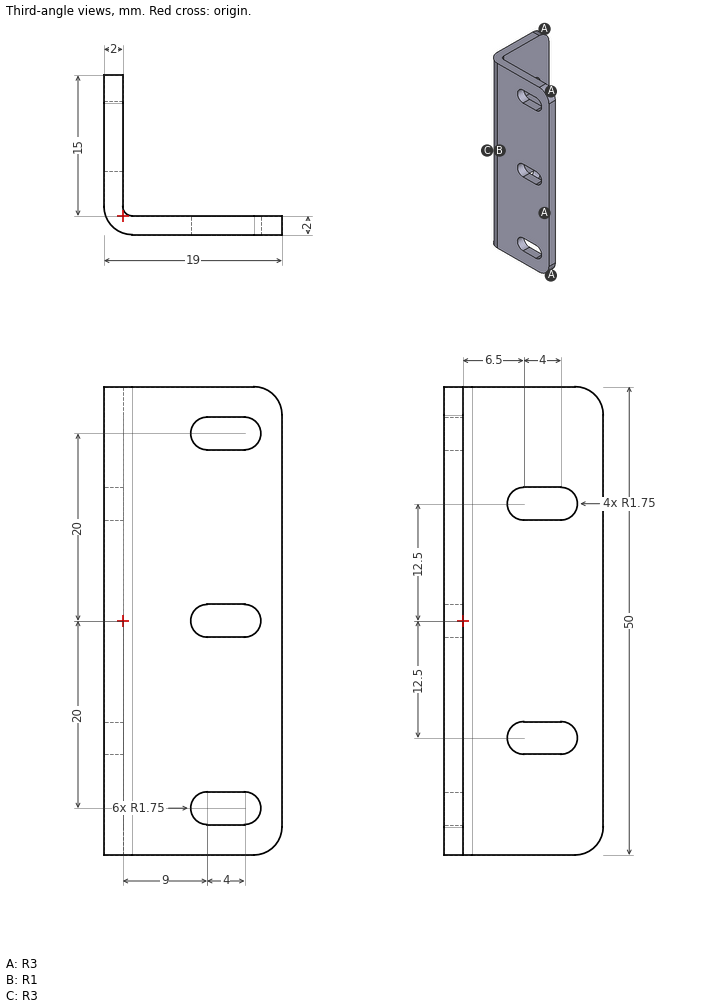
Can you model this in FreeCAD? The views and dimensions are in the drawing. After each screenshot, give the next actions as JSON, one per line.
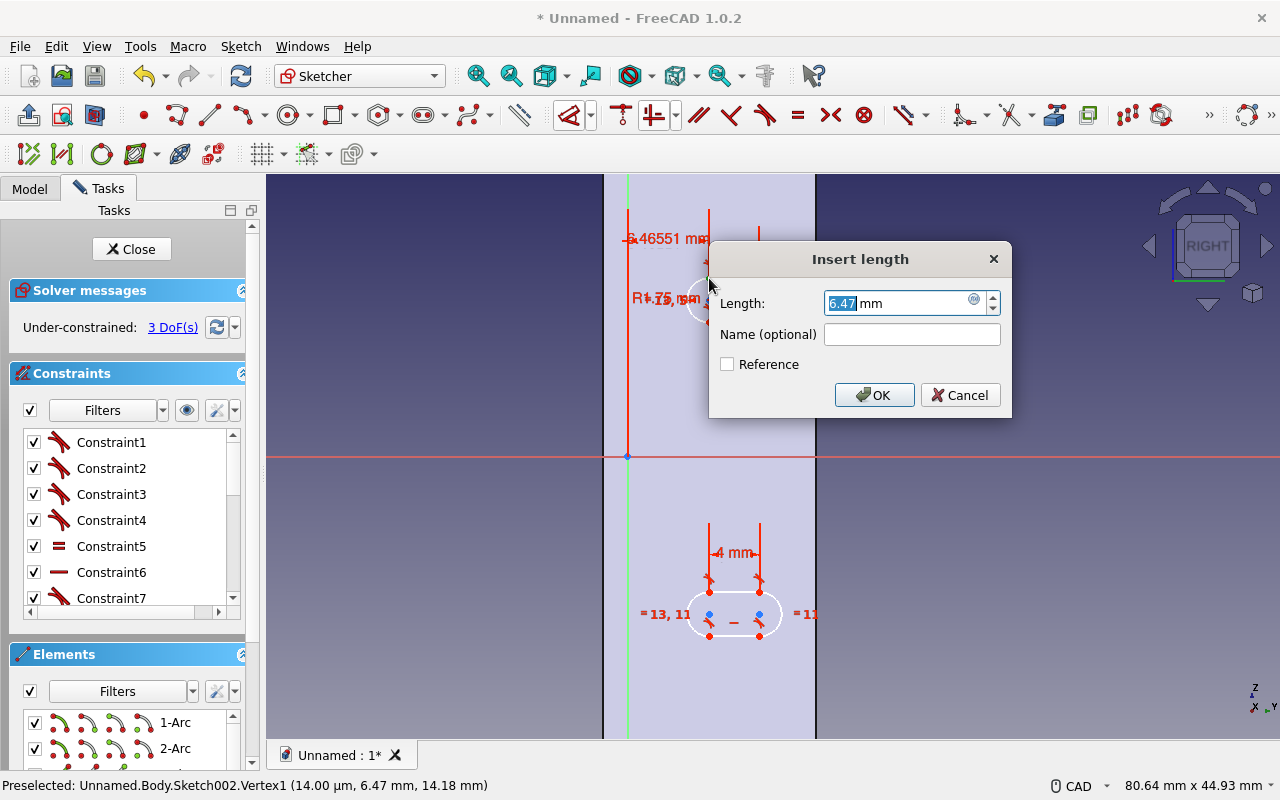
{"action": "type", "text": "6.5"}
{"action": "key", "text": "Return"}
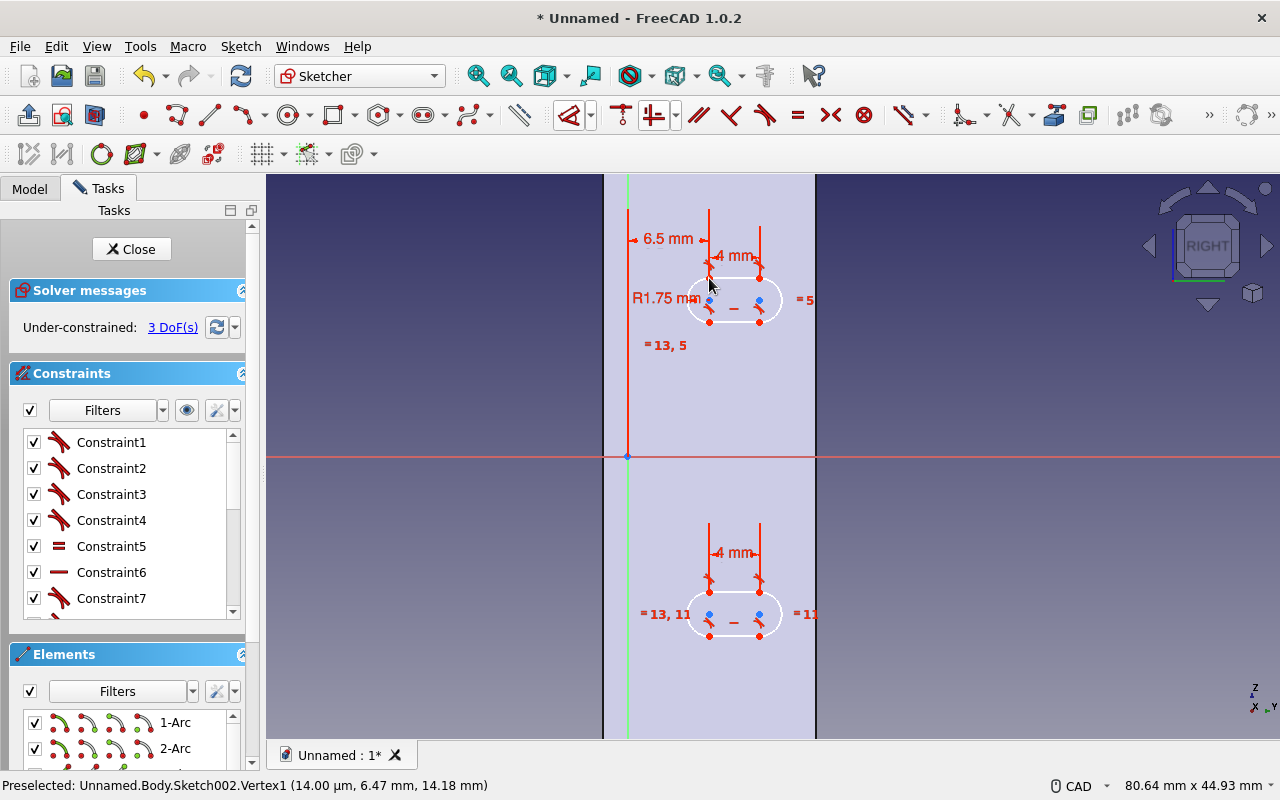
{"action": "left_click", "coordinate": [709, 592]}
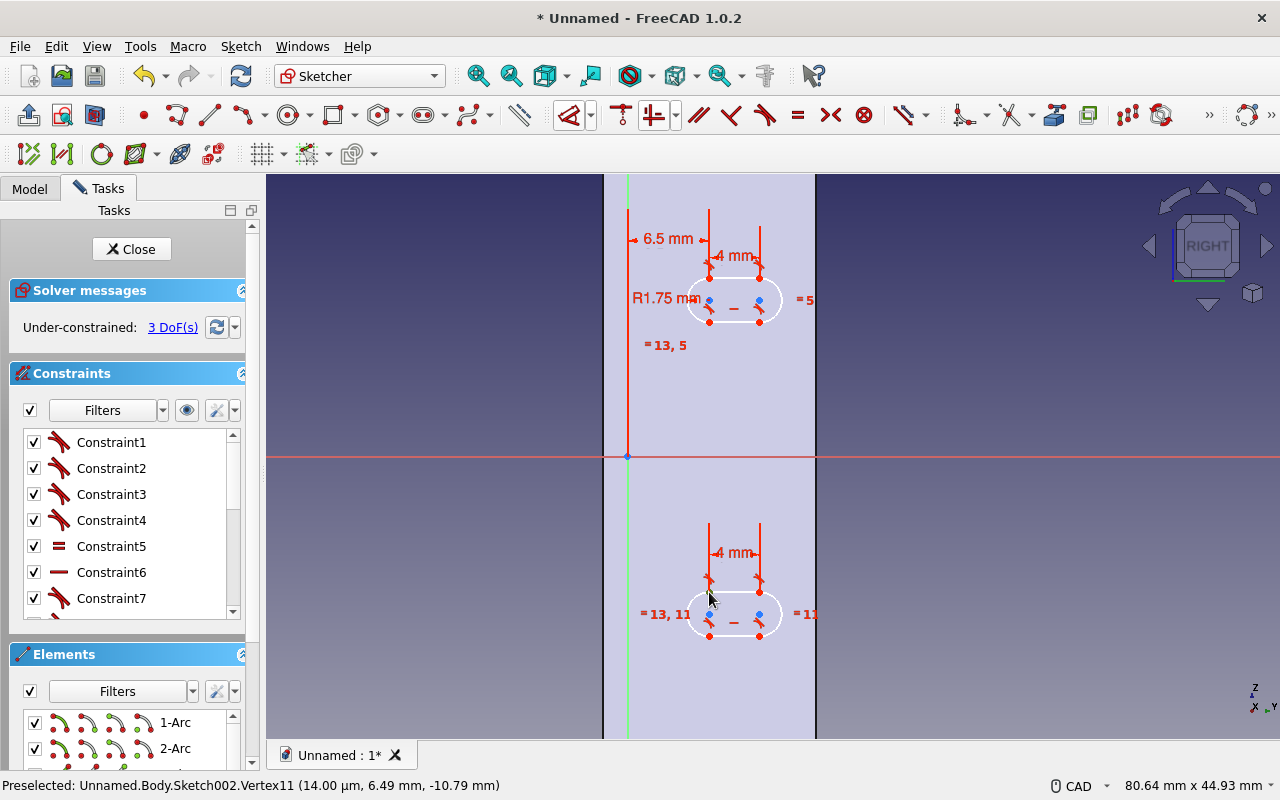
{"action": "key", "text": "l"}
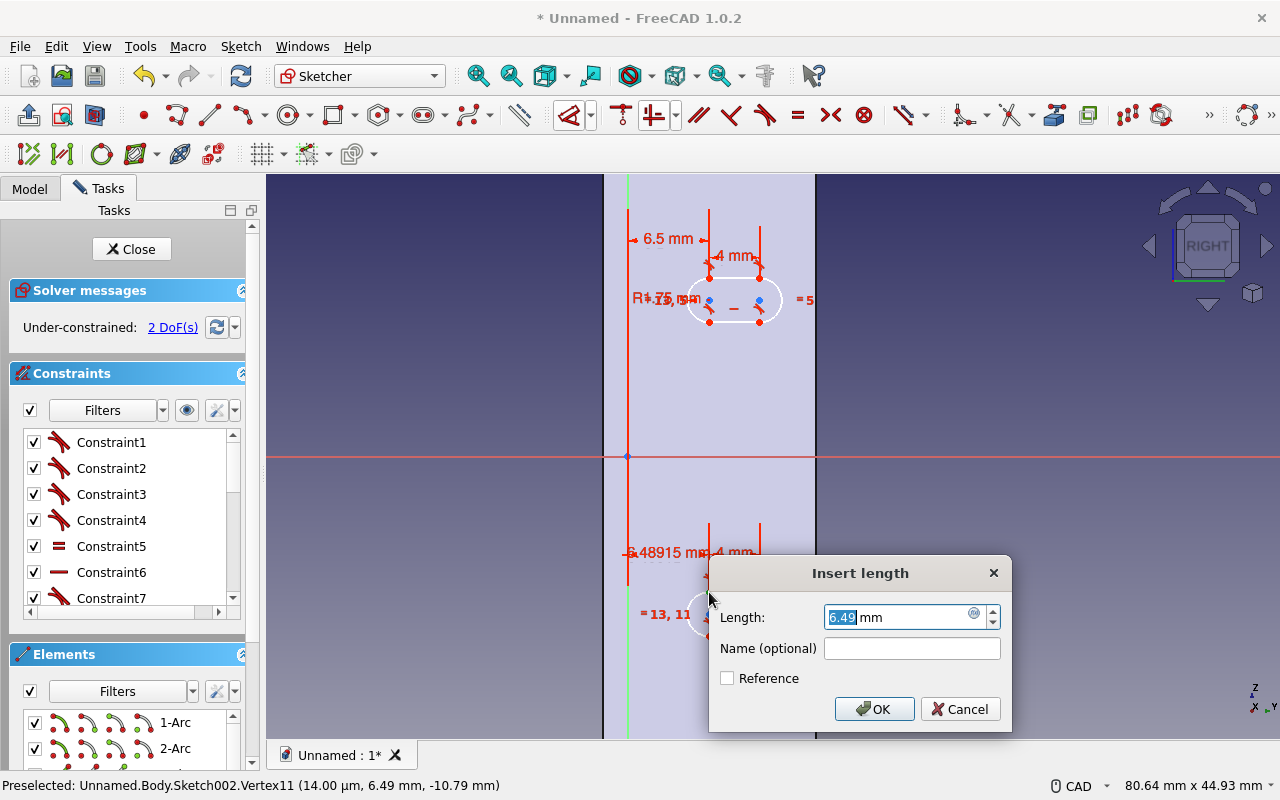
{"action": "type", "text": "6.5"}
{"action": "key", "text": "Return"}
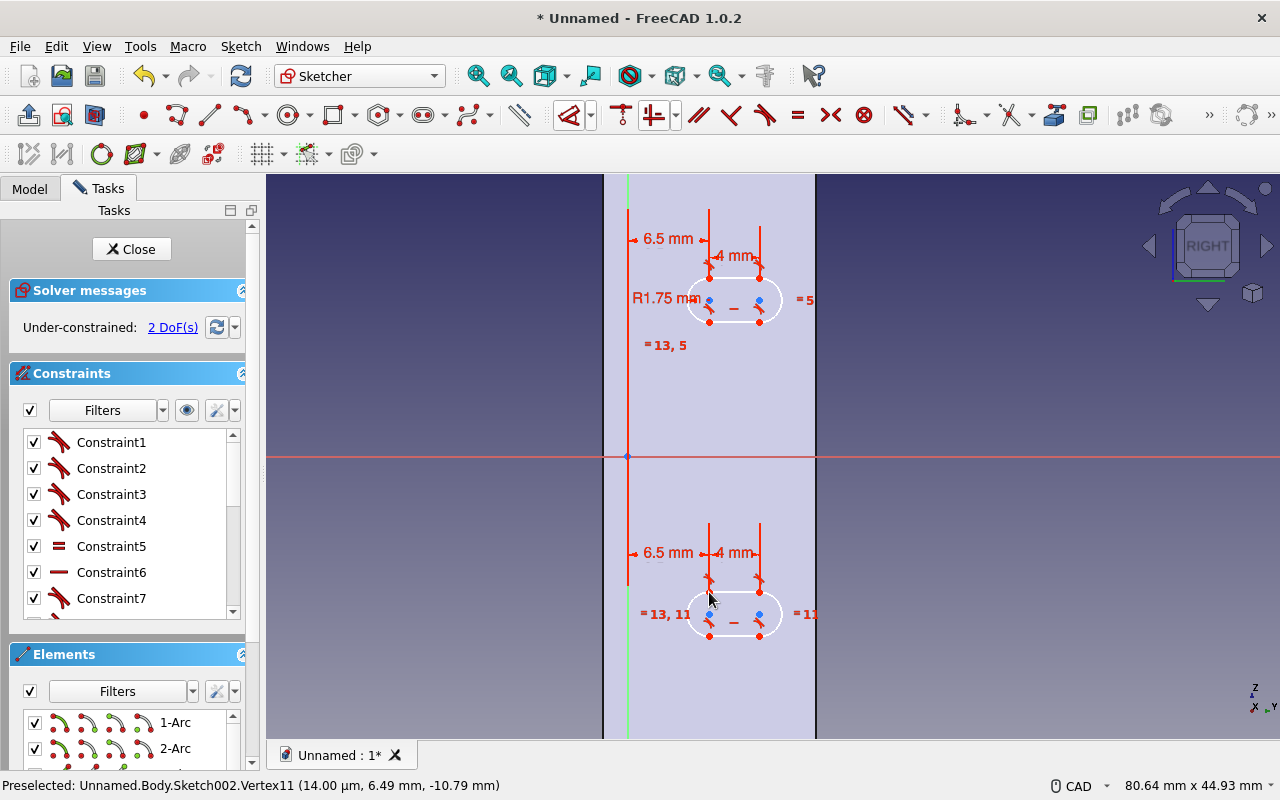
{"action": "left_click", "coordinate": [709, 300]}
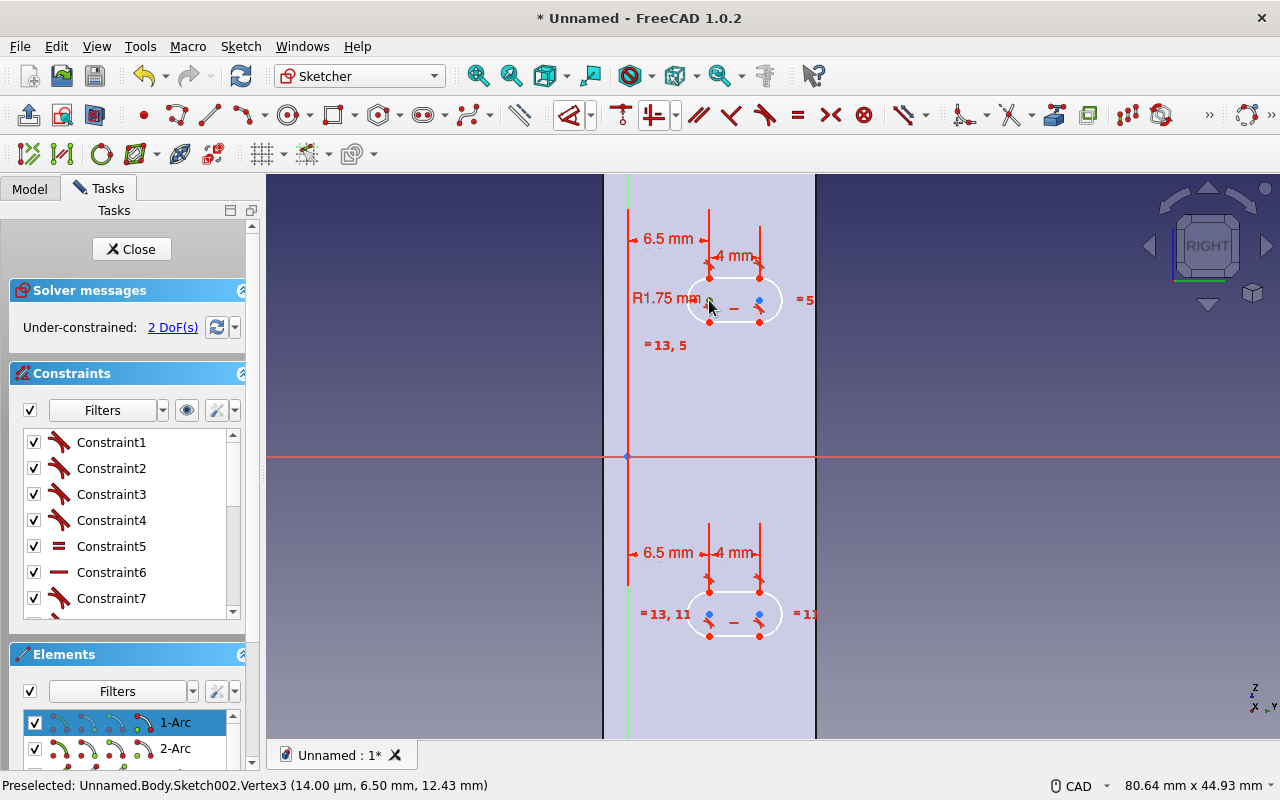
{"action": "left_click", "coordinate": [590, 116]}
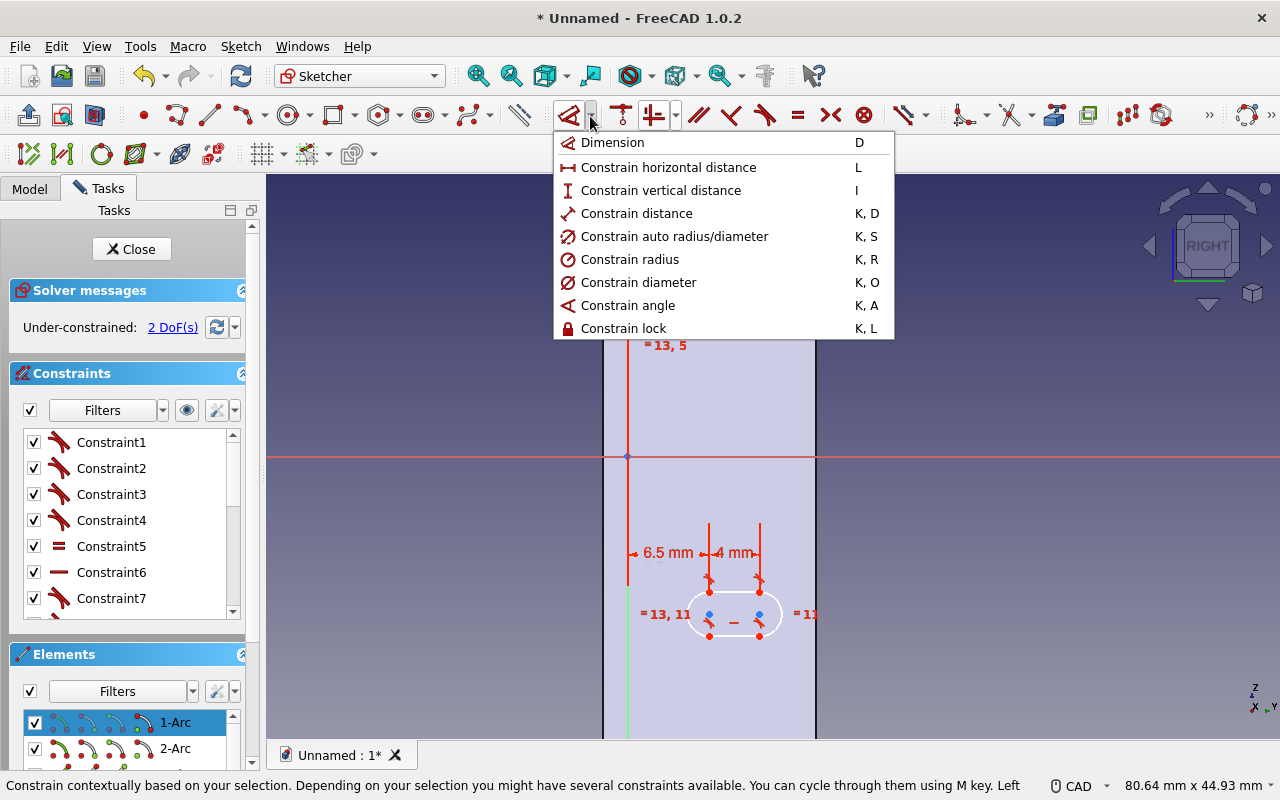
{"action": "left_click", "coordinate": [724, 190]}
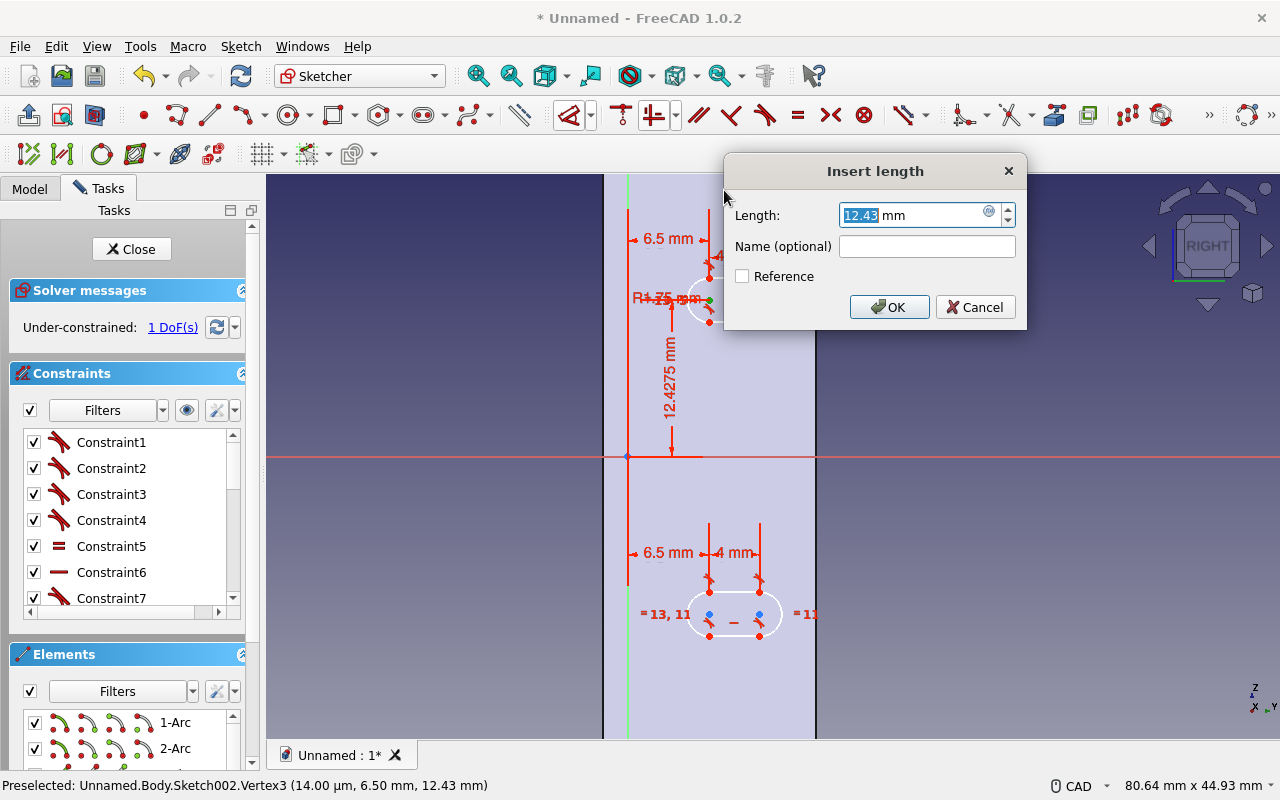
{"action": "type", "text": "12.5"}
{"action": "key", "text": "Return"}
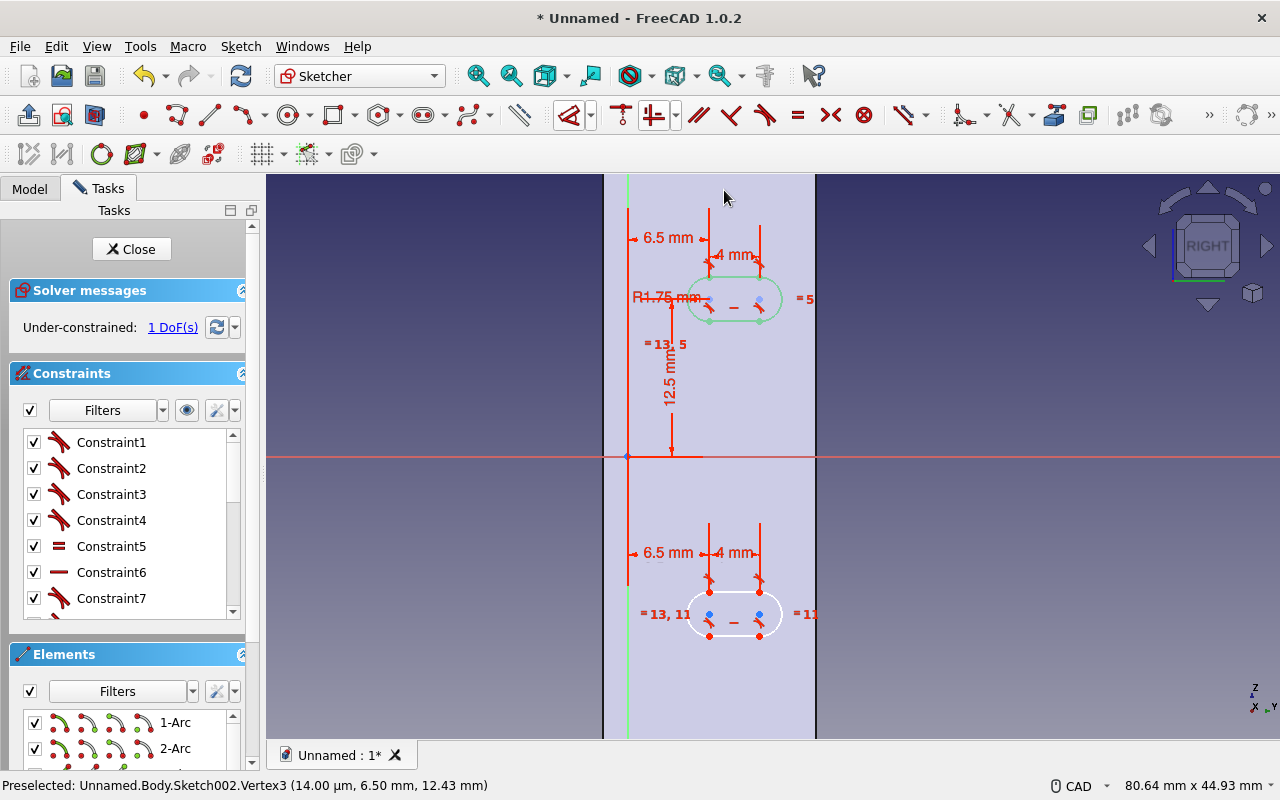
{"action": "left_click", "coordinate": [709, 614]}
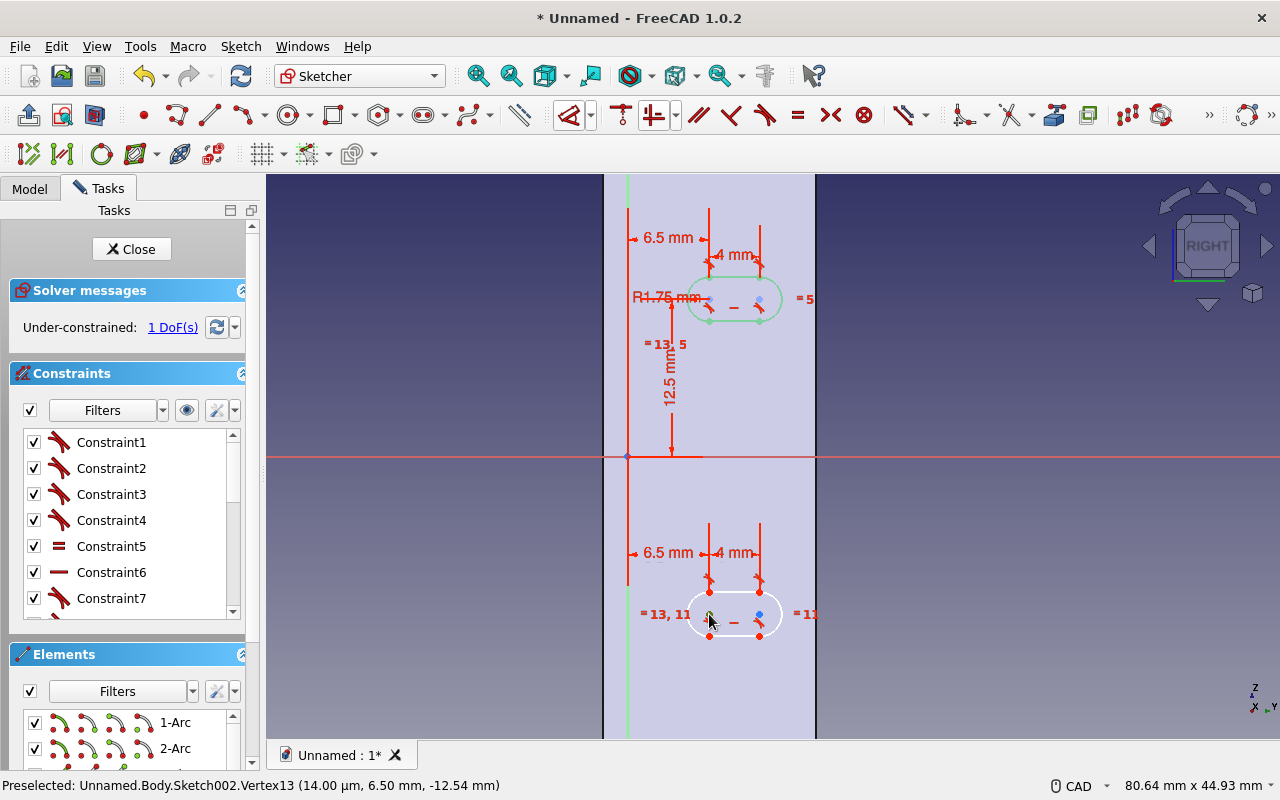
{"action": "left_click", "coordinate": [590, 116]}